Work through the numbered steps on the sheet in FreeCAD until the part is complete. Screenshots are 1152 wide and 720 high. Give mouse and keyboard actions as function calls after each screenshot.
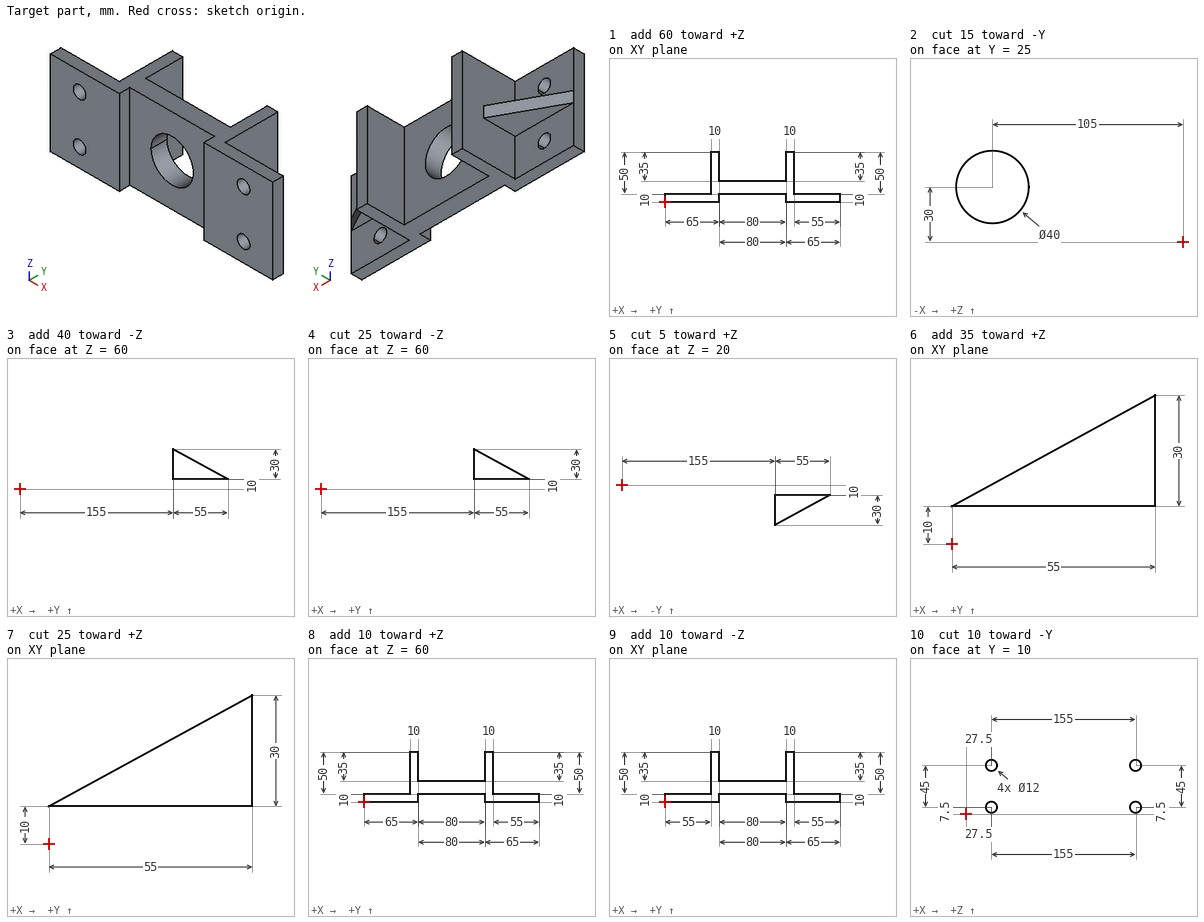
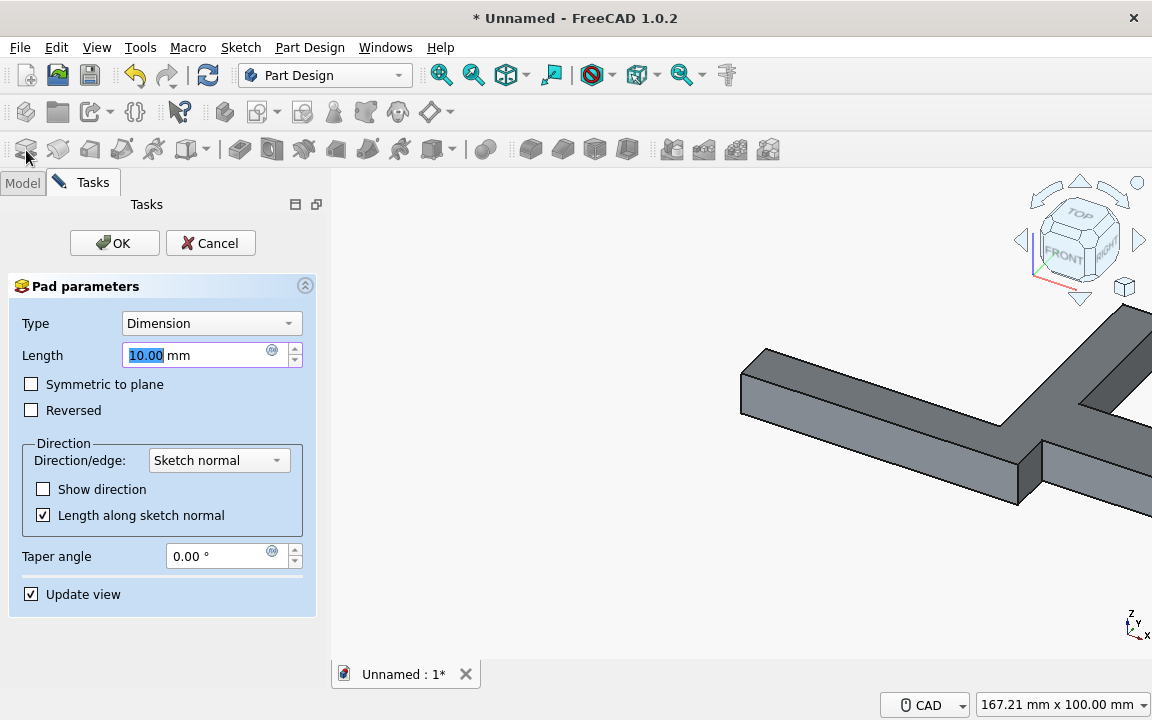
text(60)
key(Tab)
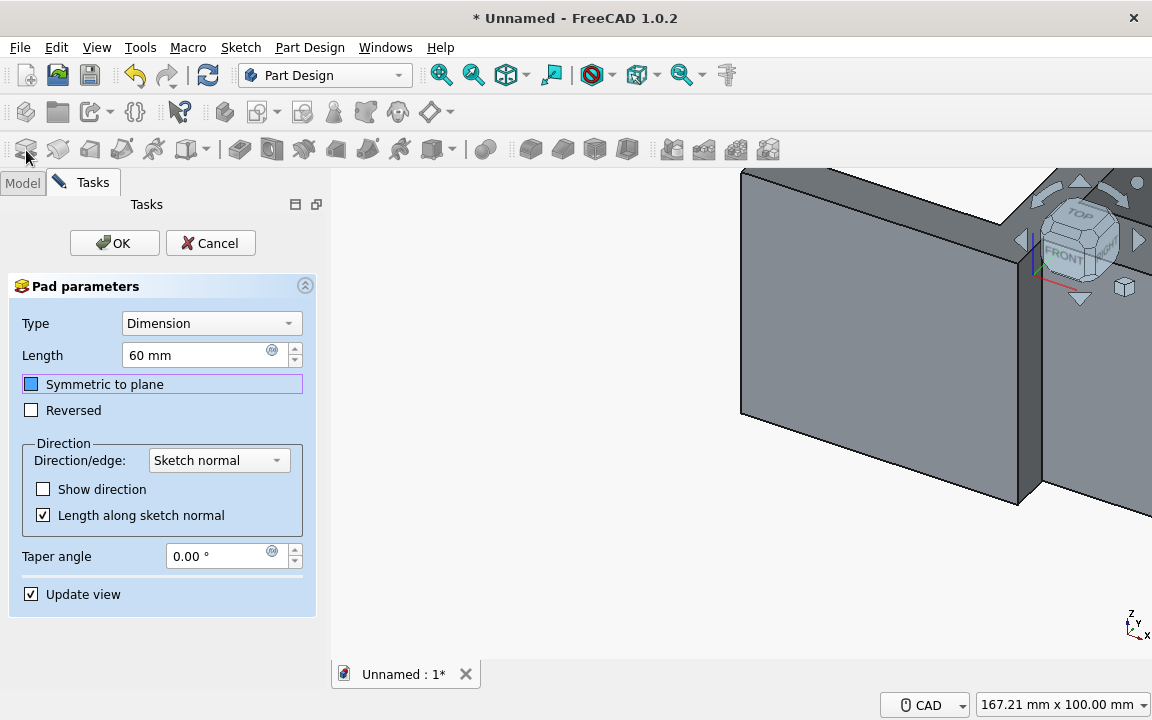
click(115, 243)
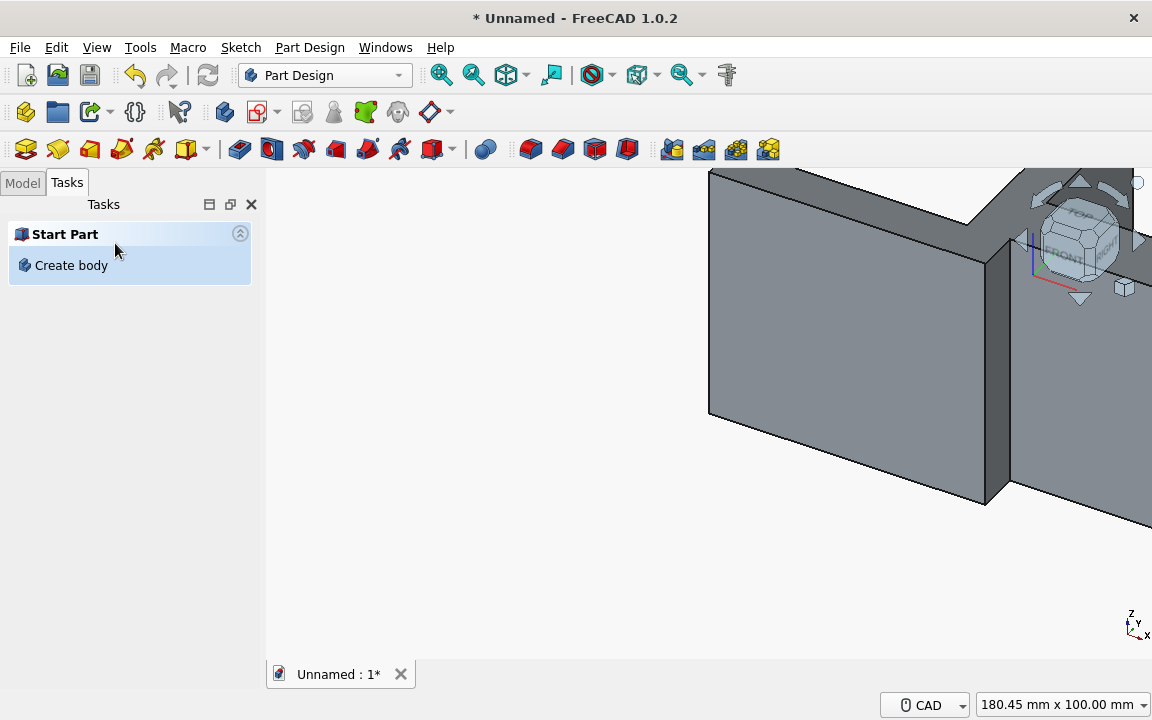
key(v)
key(f)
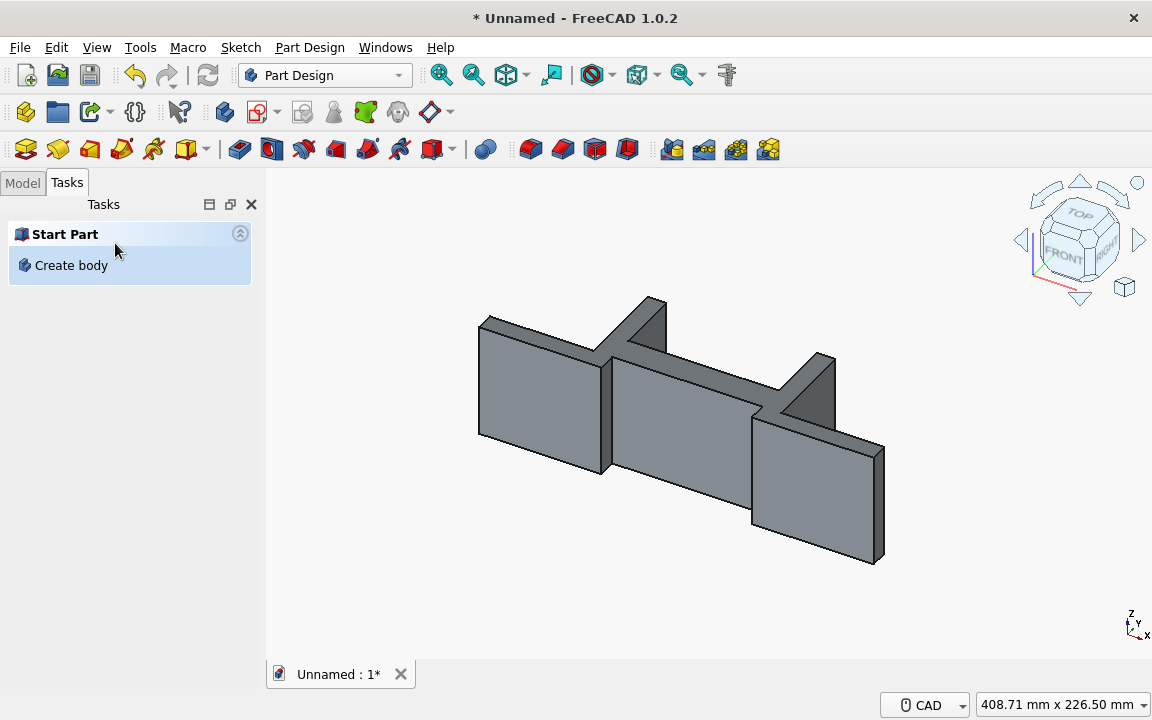
key(4)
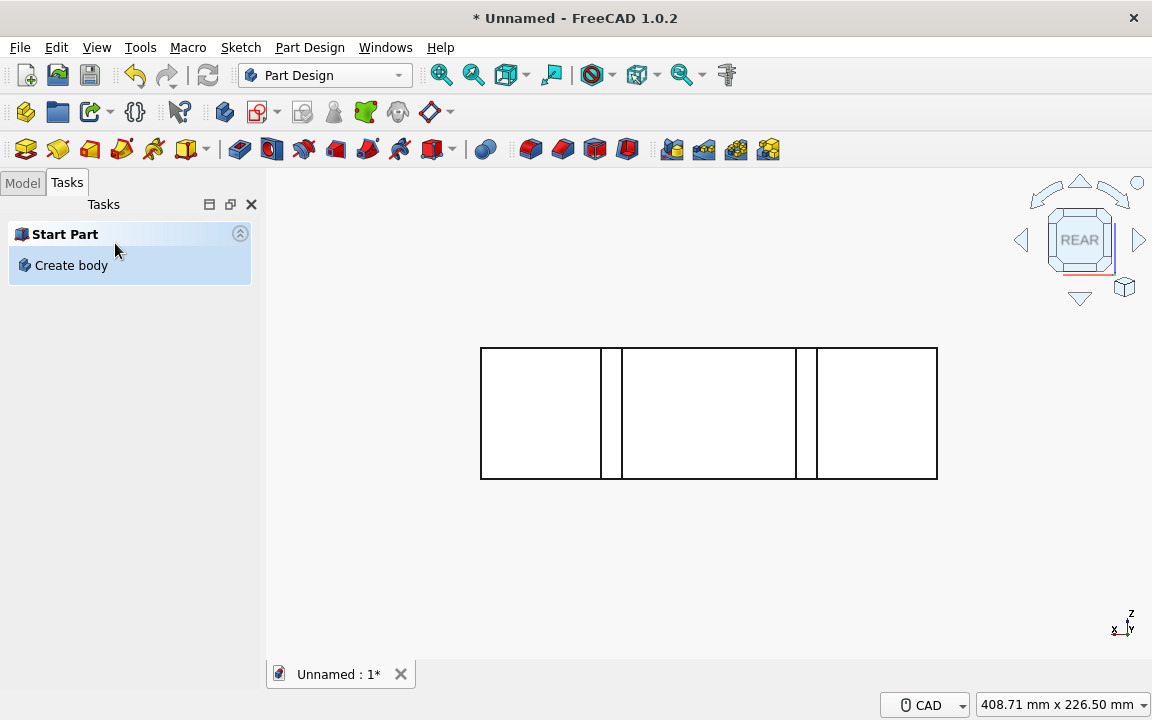
click(709, 413)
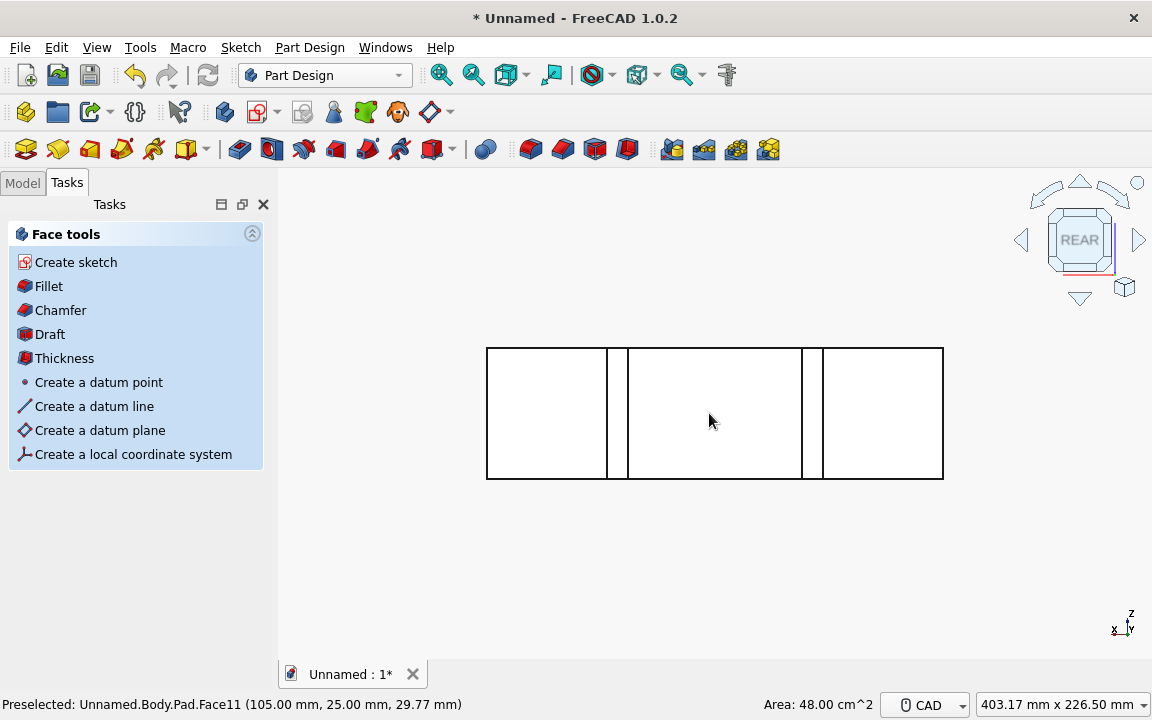
click(258, 112)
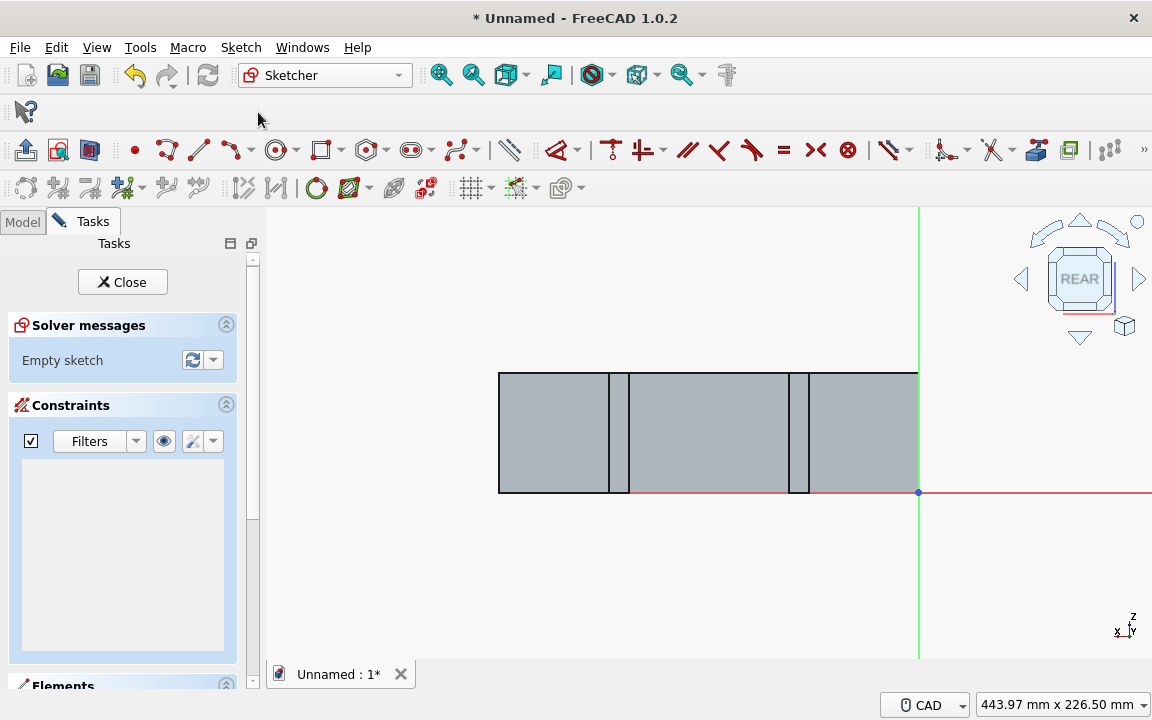
click(90, 150)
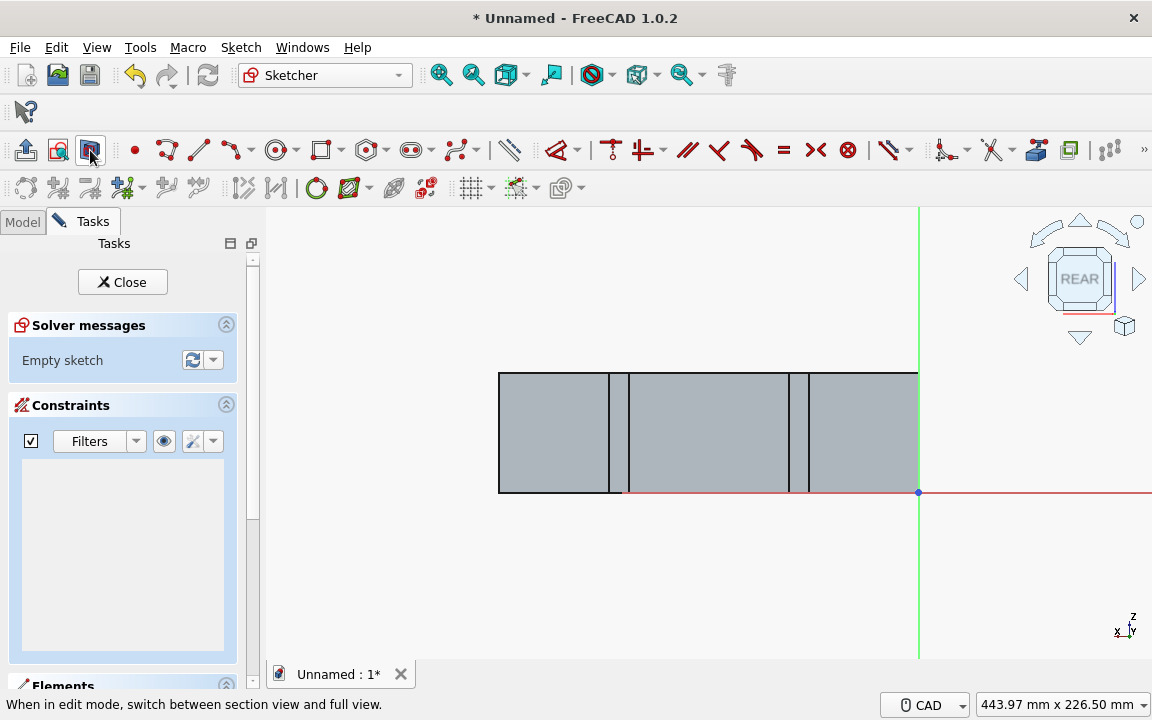
scroll(739, 433, up, 6)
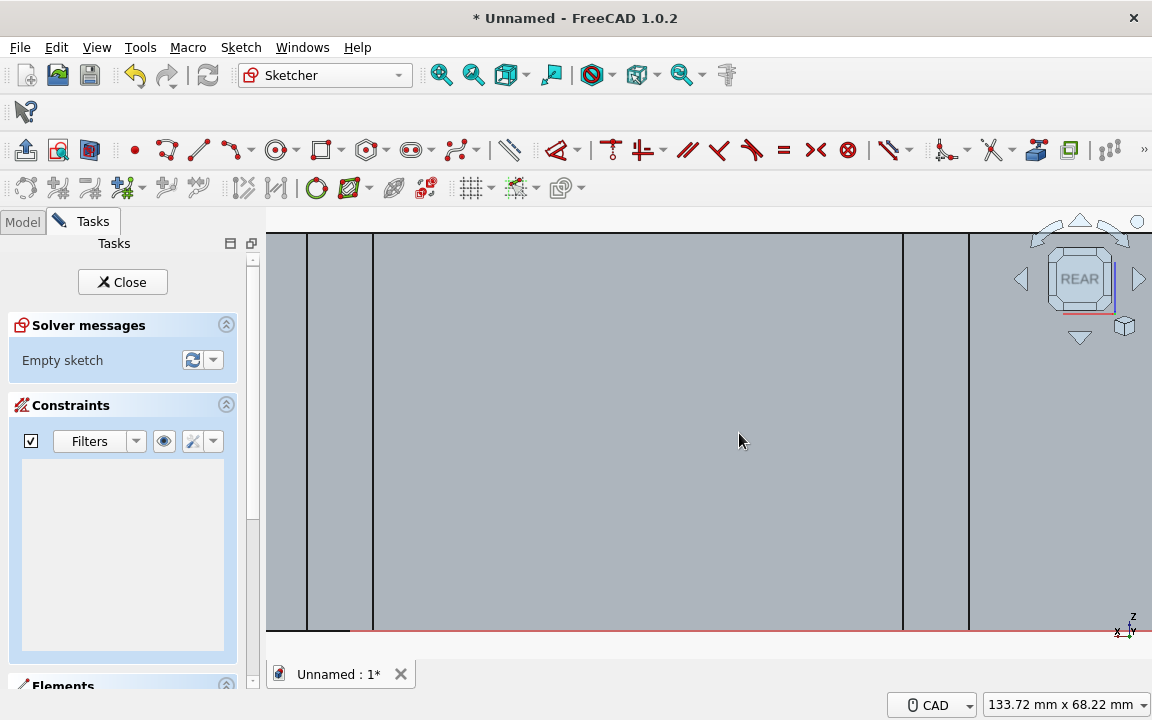
click(276, 150)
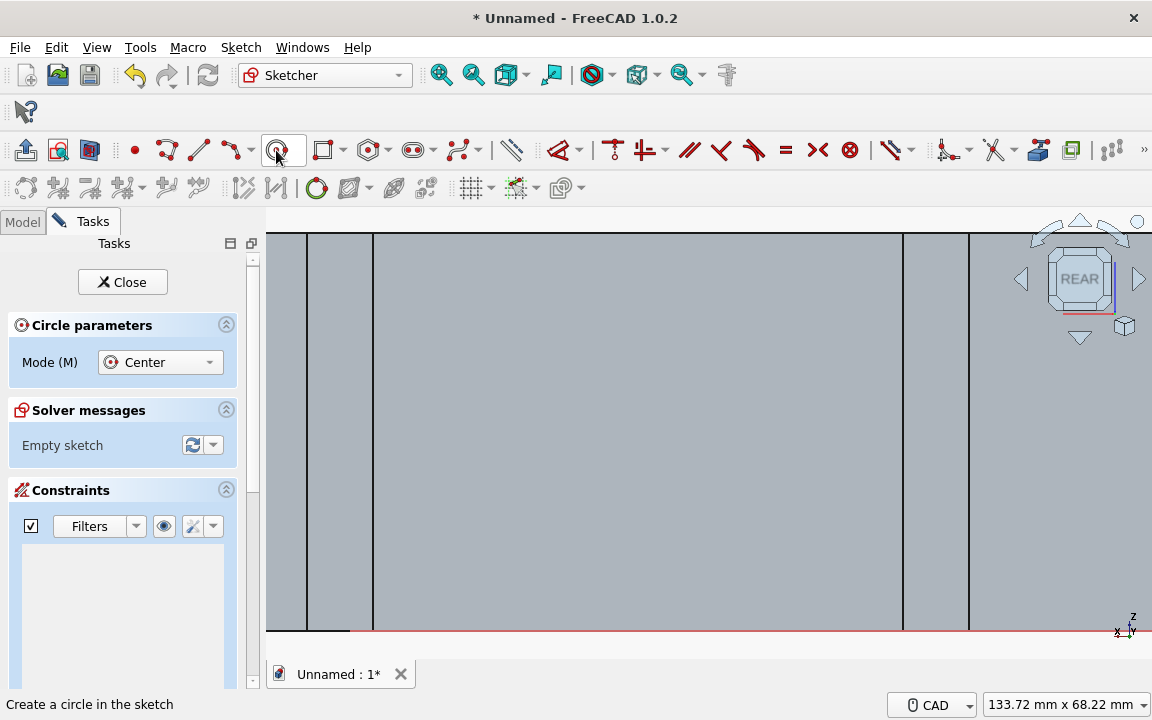
click(638, 432)
move(732, 338)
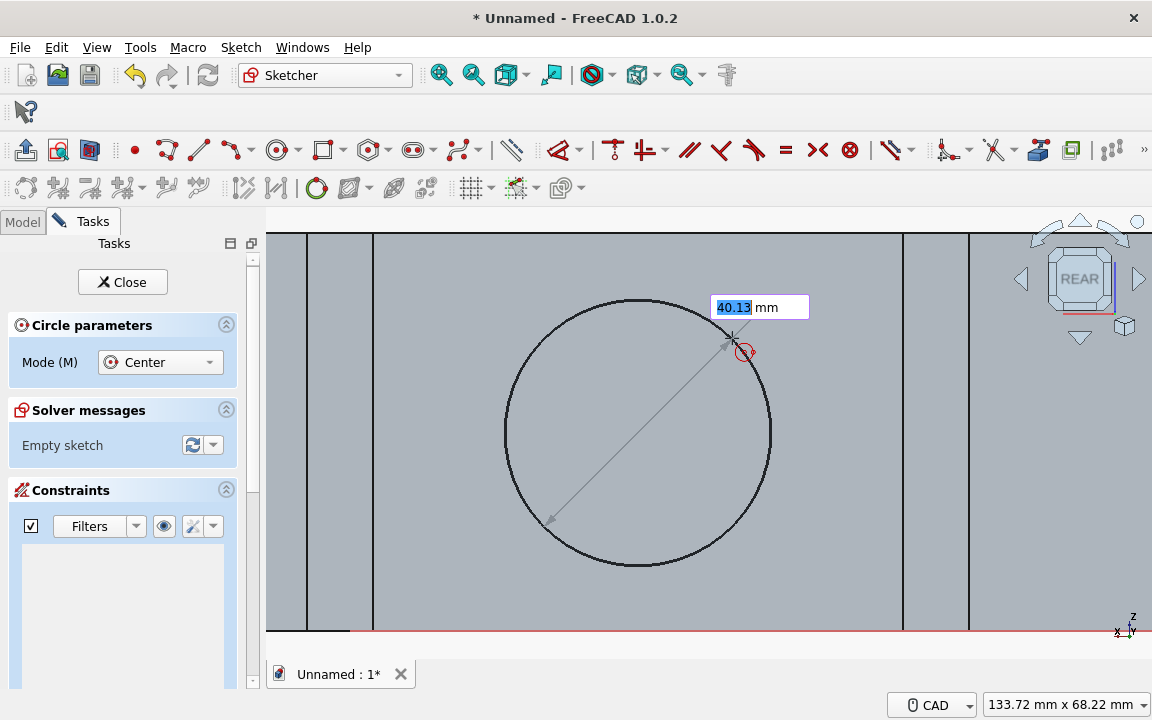
text(40)
key(Return)
key(Escape)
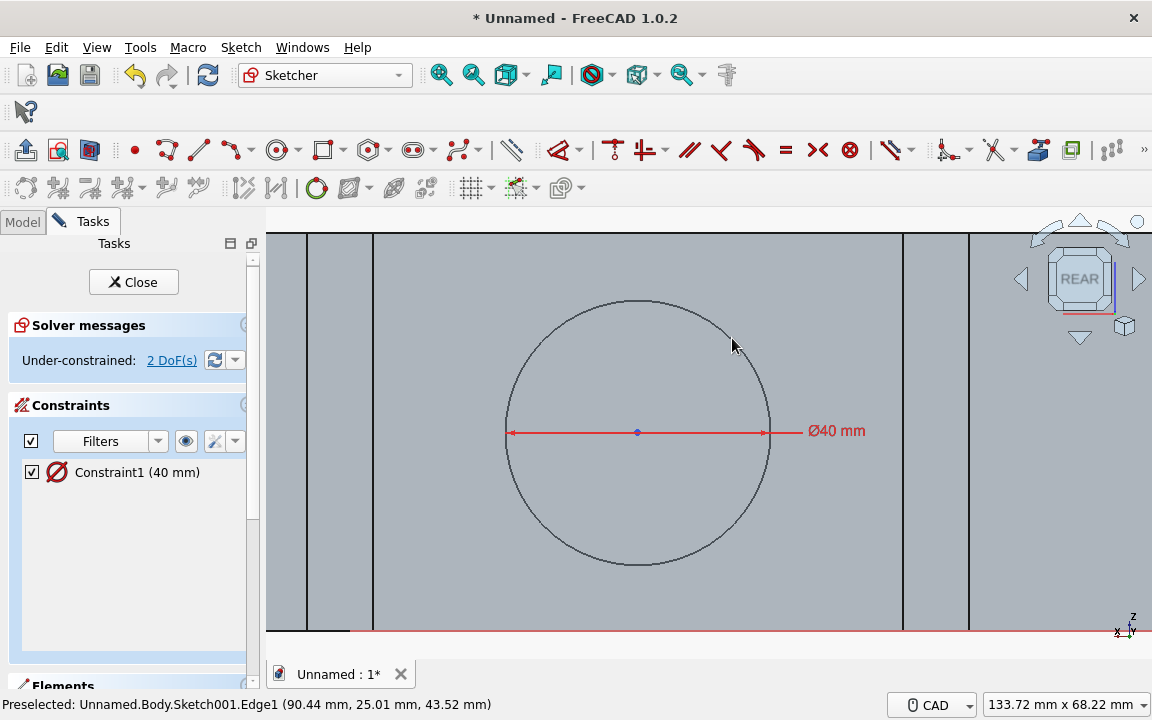
key(d)